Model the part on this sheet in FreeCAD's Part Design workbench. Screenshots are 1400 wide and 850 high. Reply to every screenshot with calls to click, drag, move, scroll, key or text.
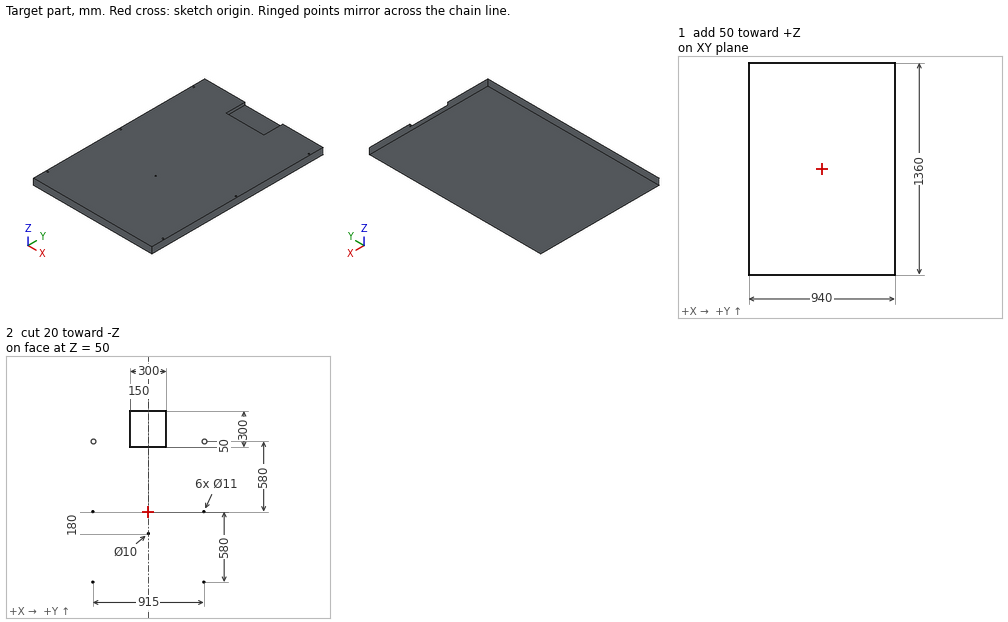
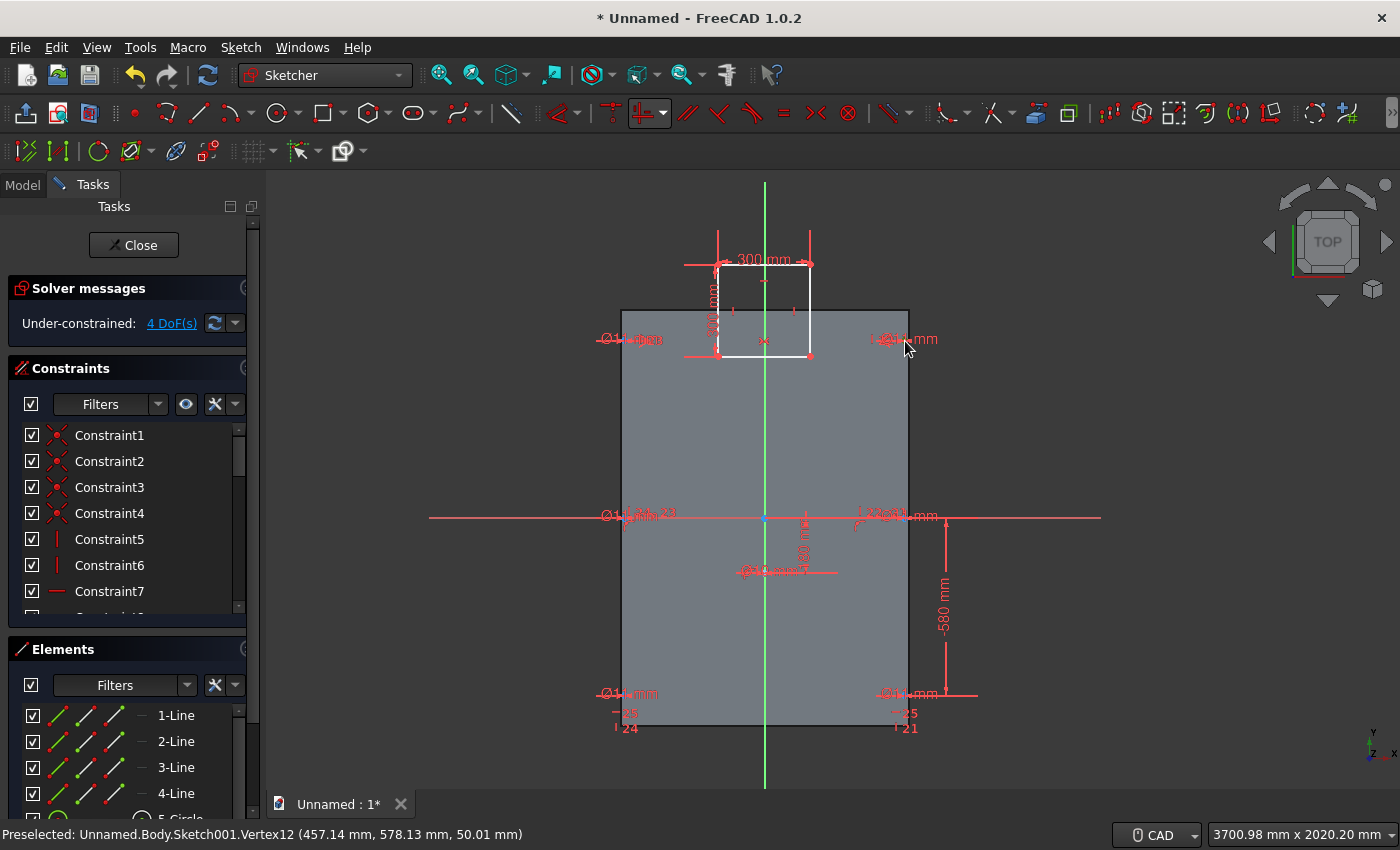
click(580, 114)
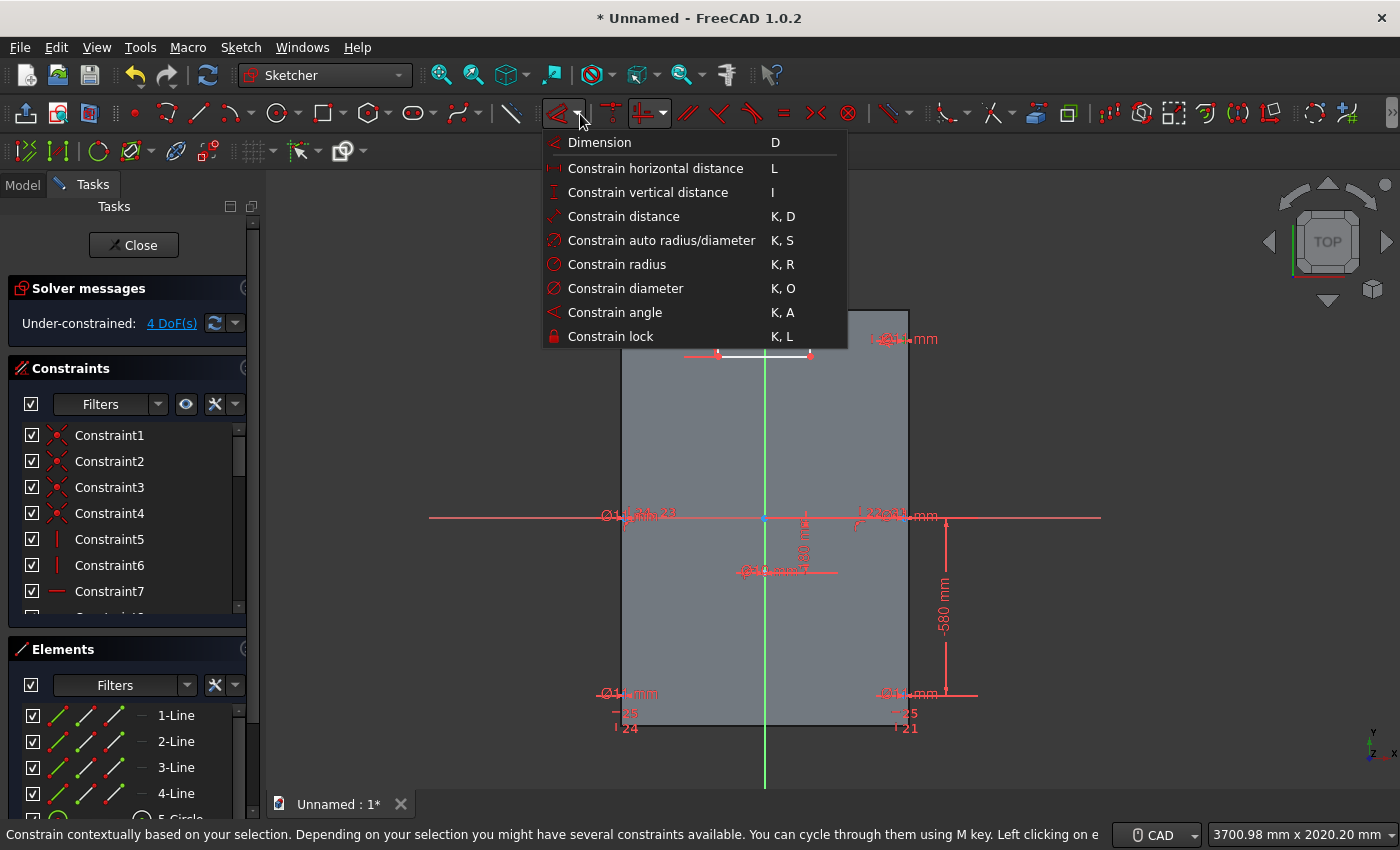
click(695, 192)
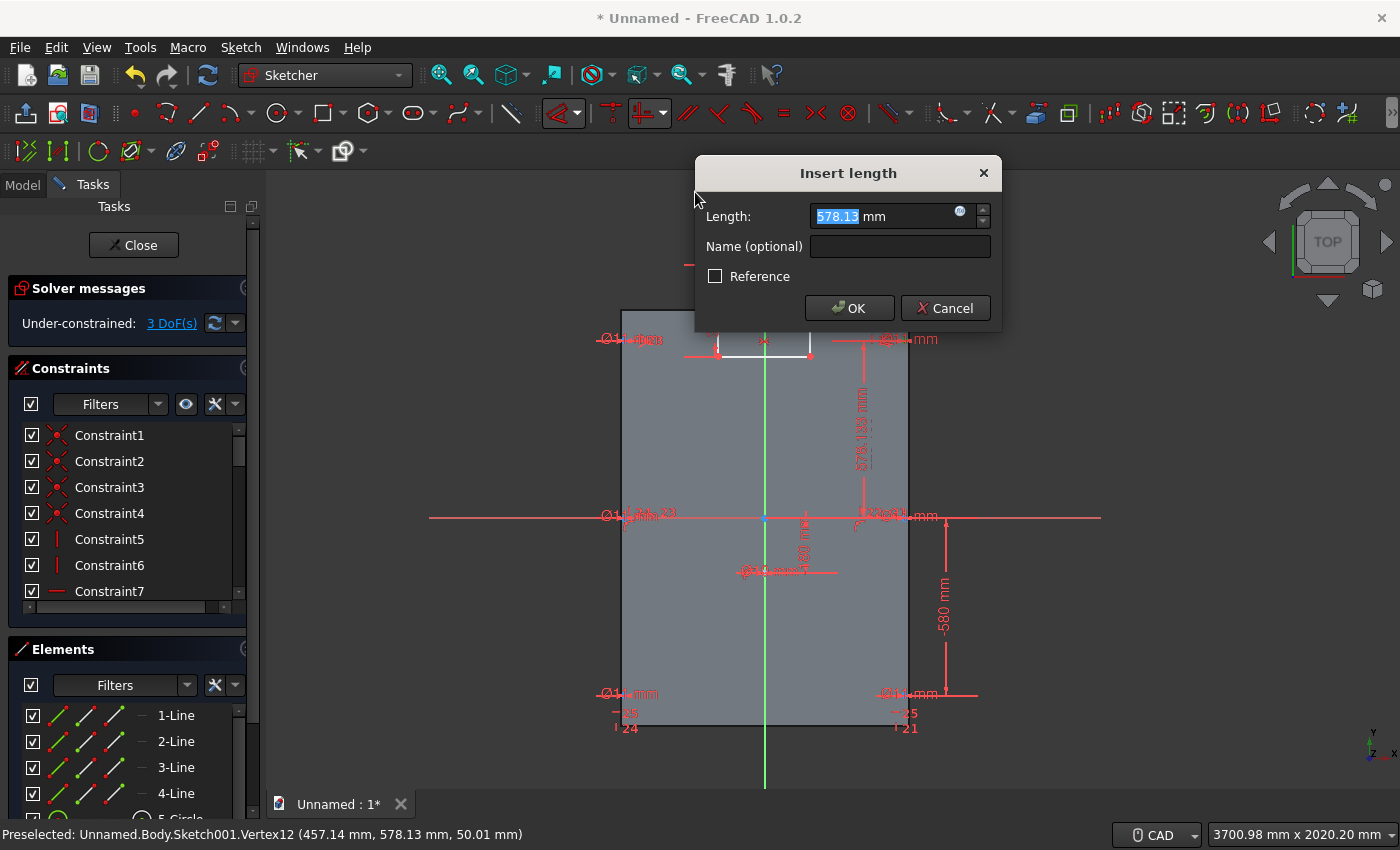
text(580)
key(Return)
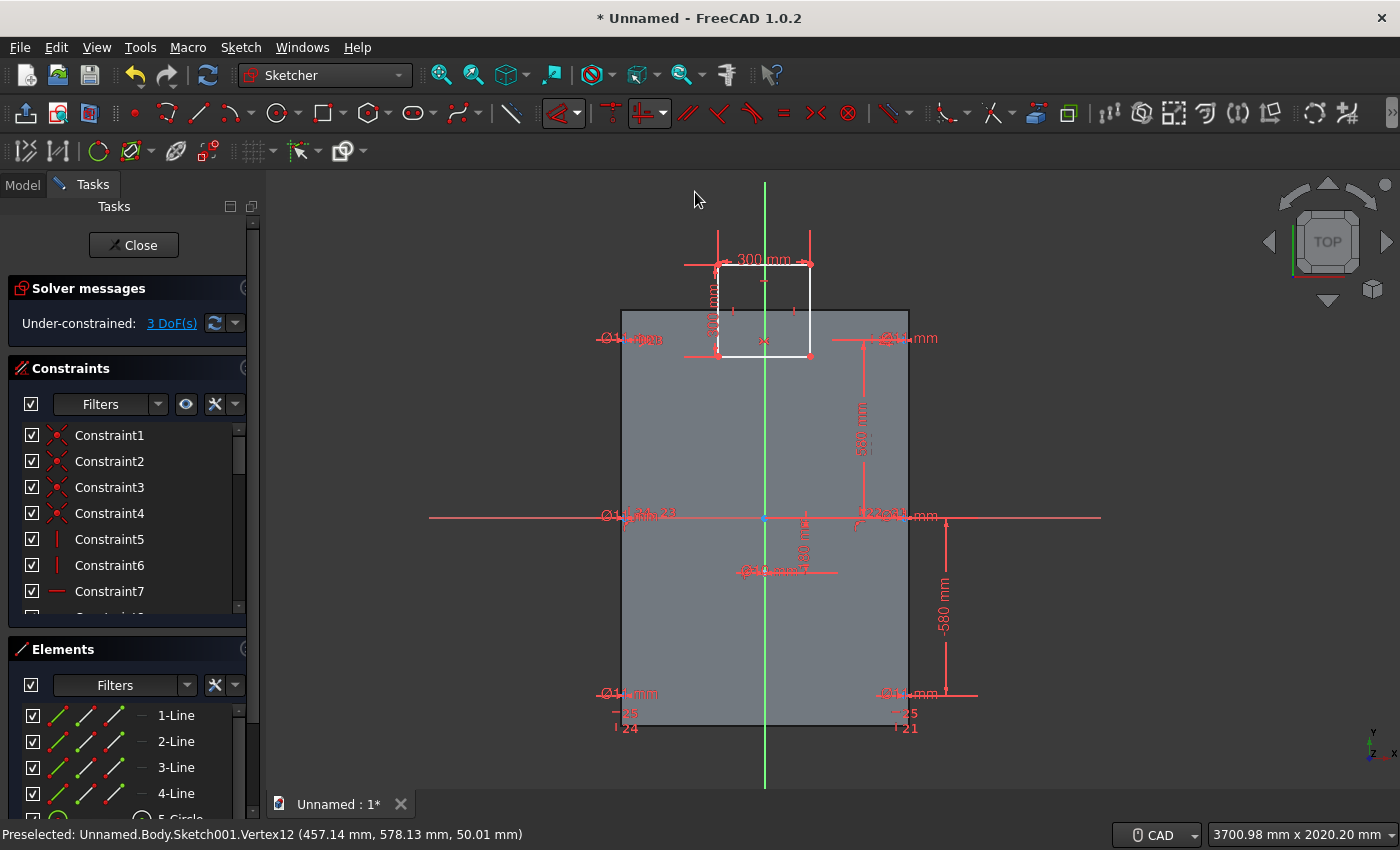
scroll(810, 357, up, 5)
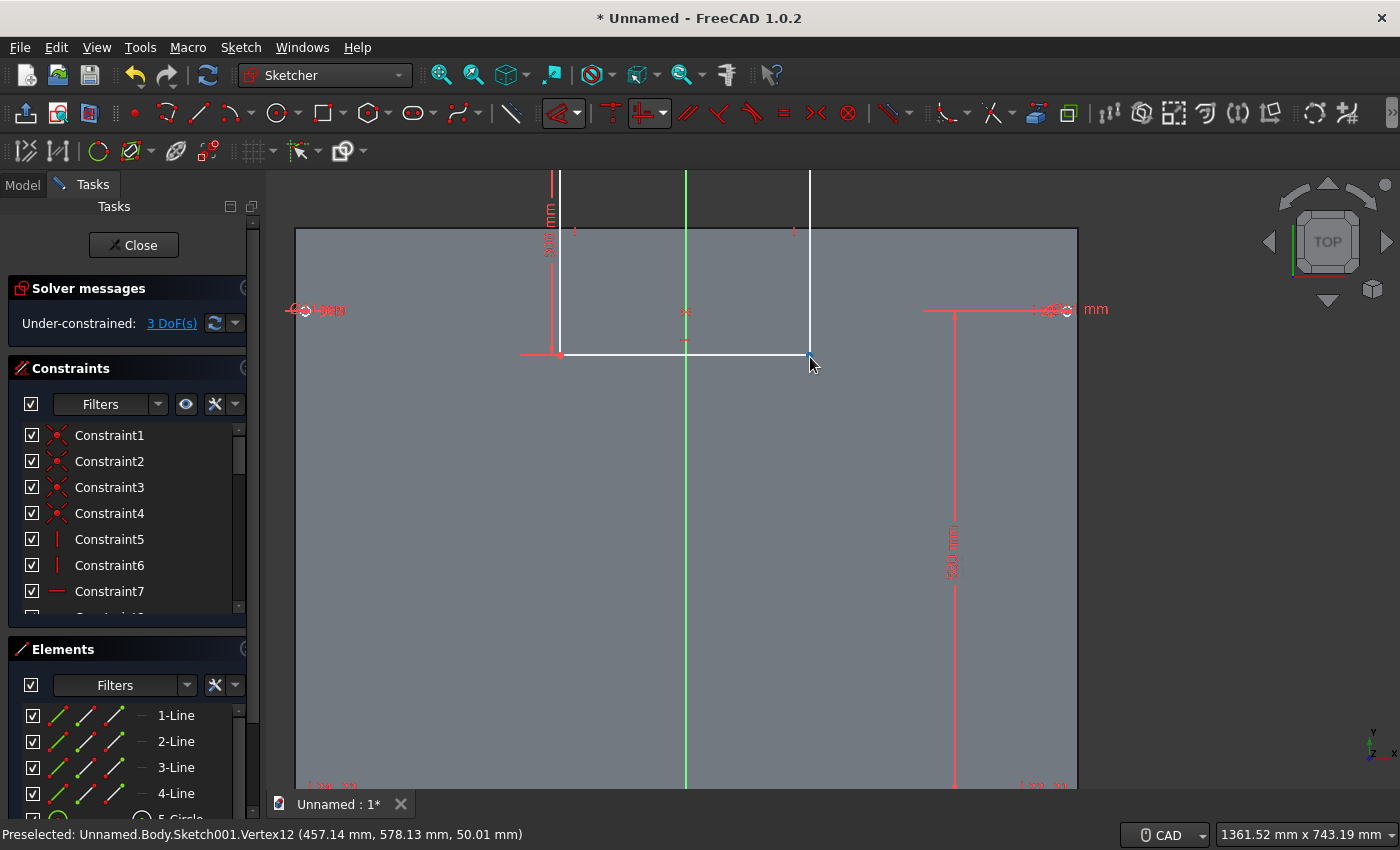
click(810, 355)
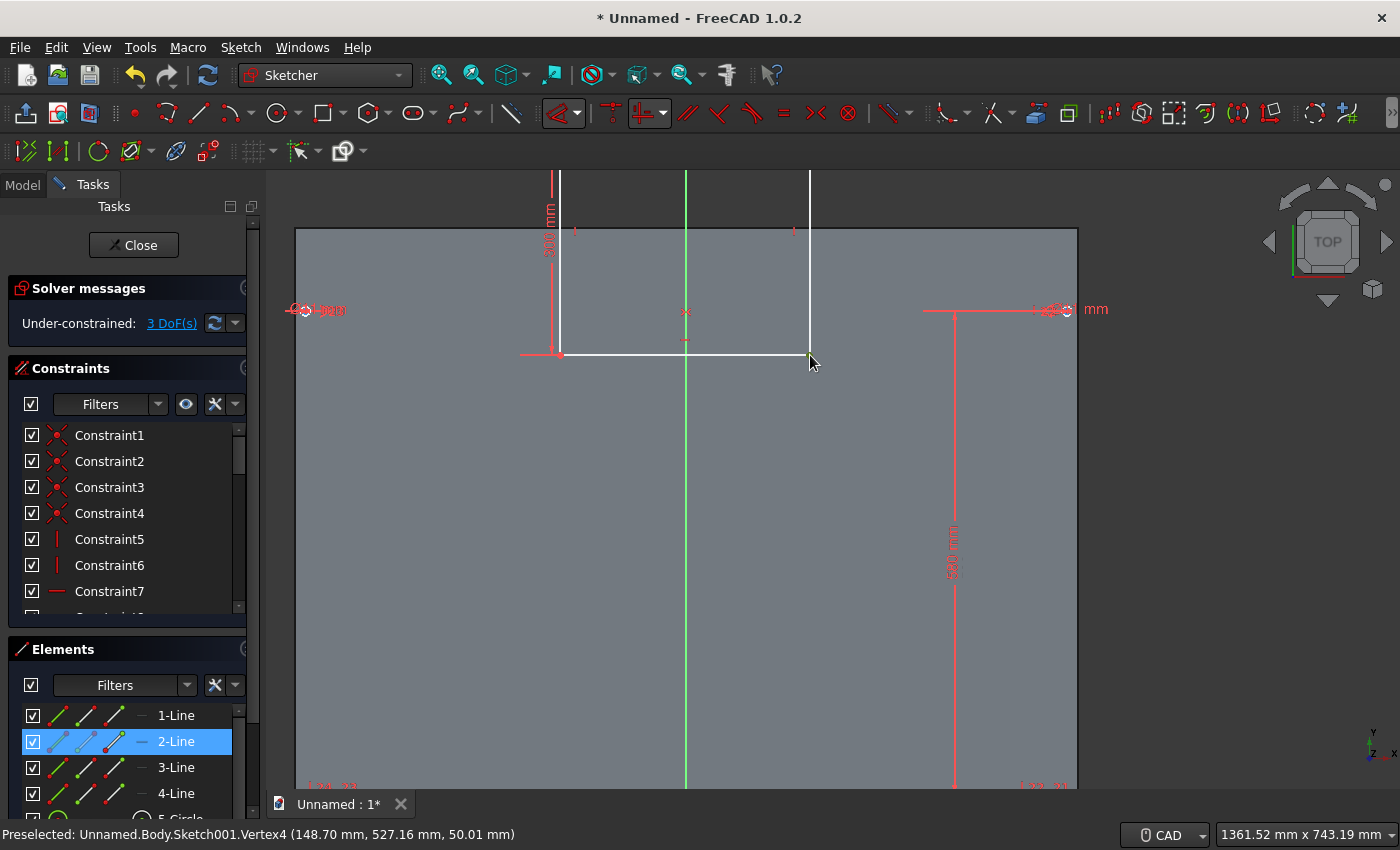
click(1067, 311)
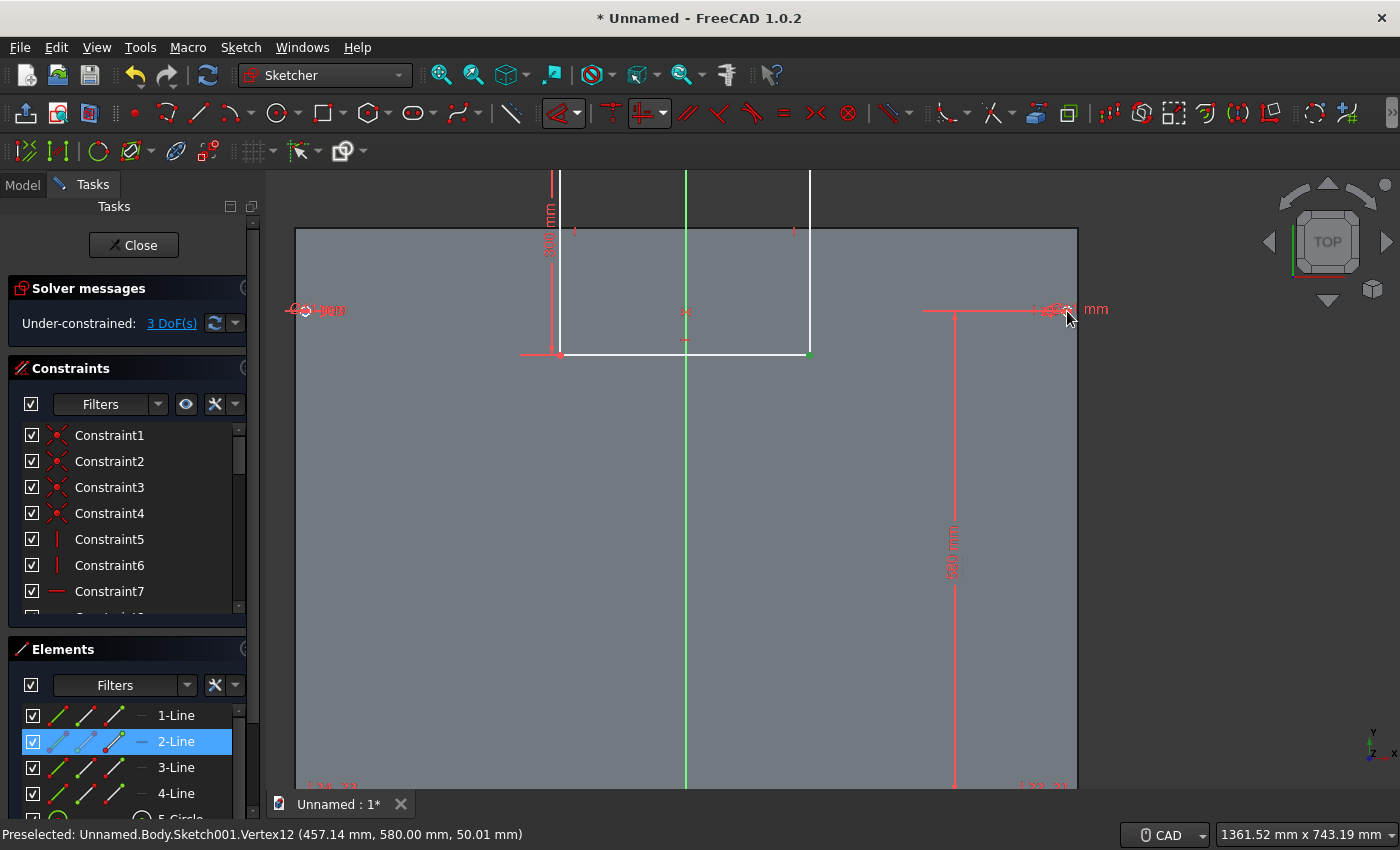
key(i)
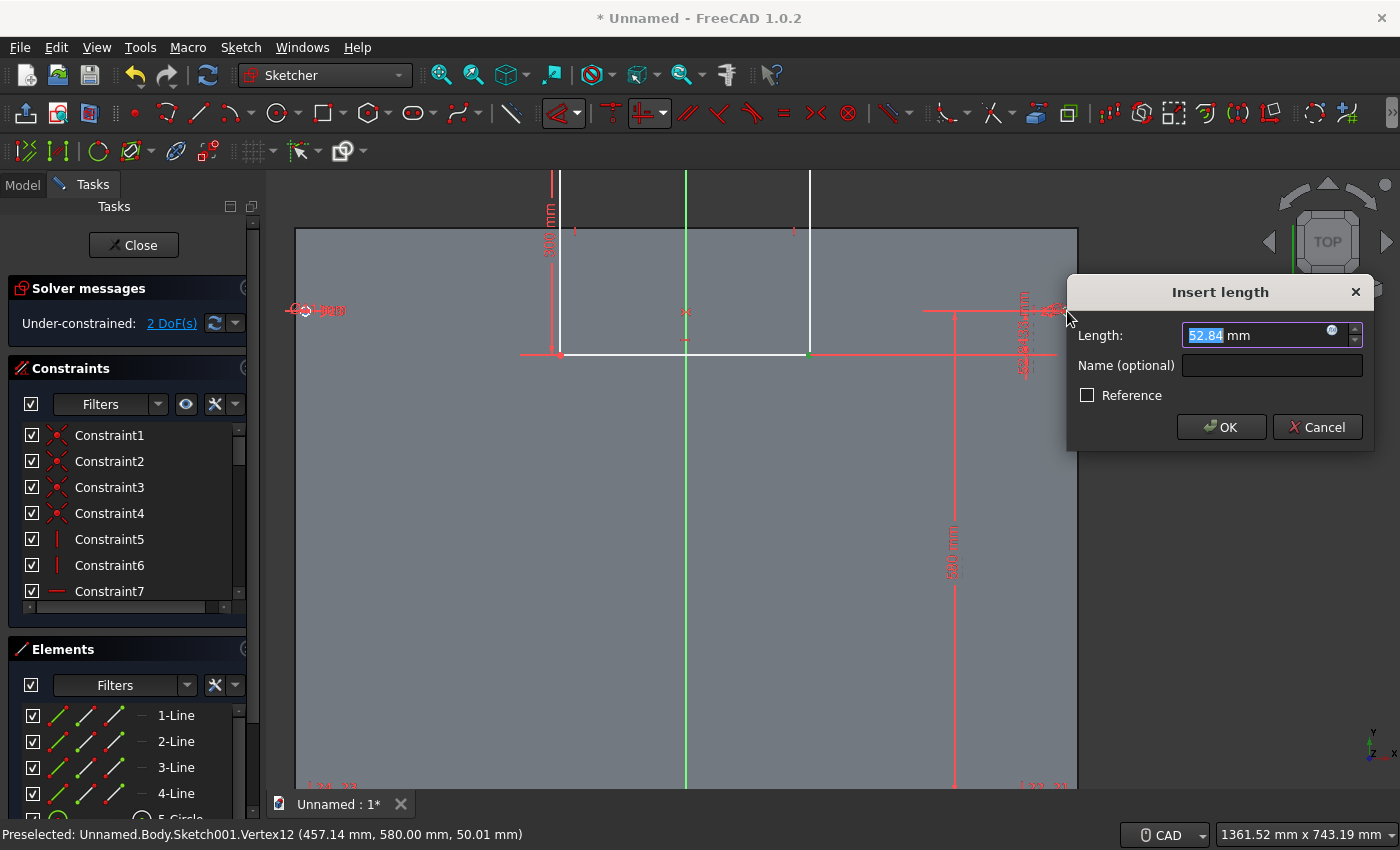
text(50)
key(Return)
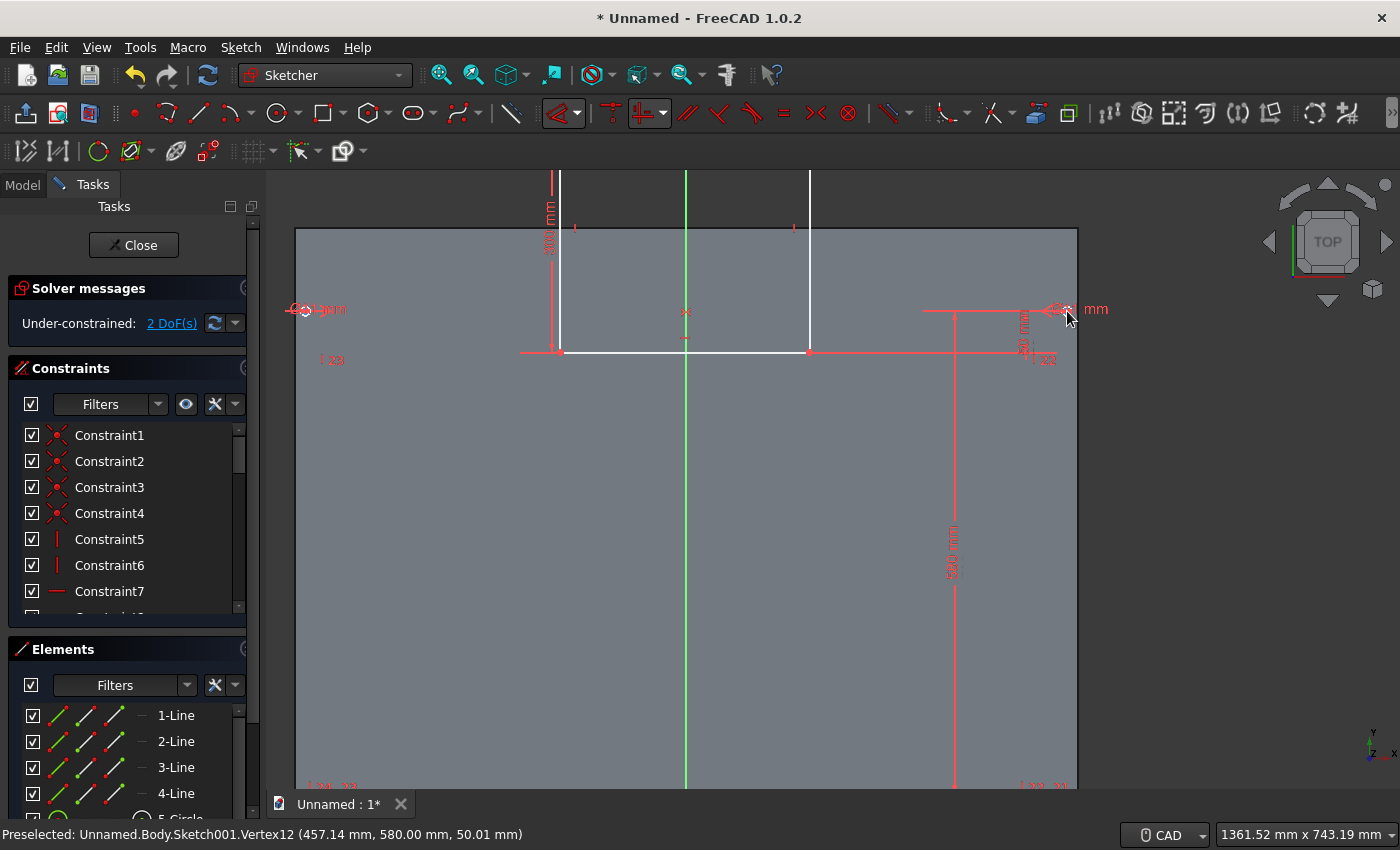
scroll(810, 356, down, 5)